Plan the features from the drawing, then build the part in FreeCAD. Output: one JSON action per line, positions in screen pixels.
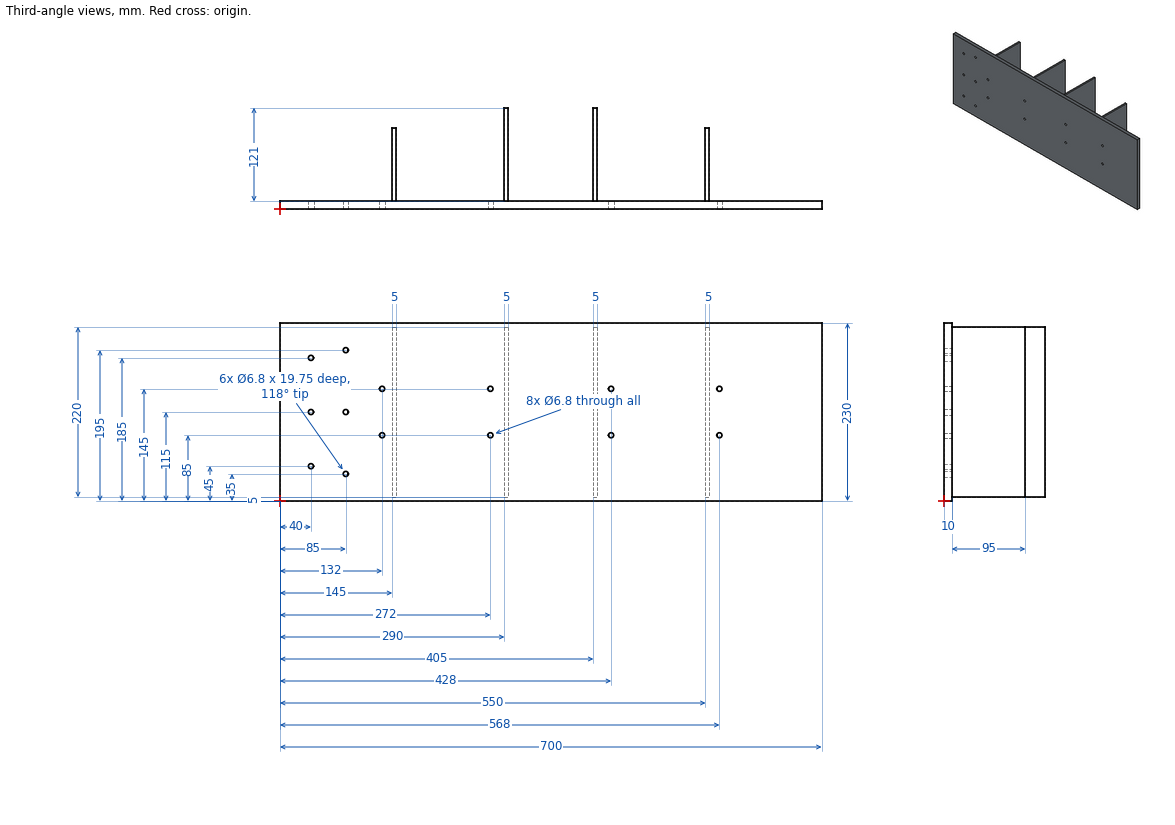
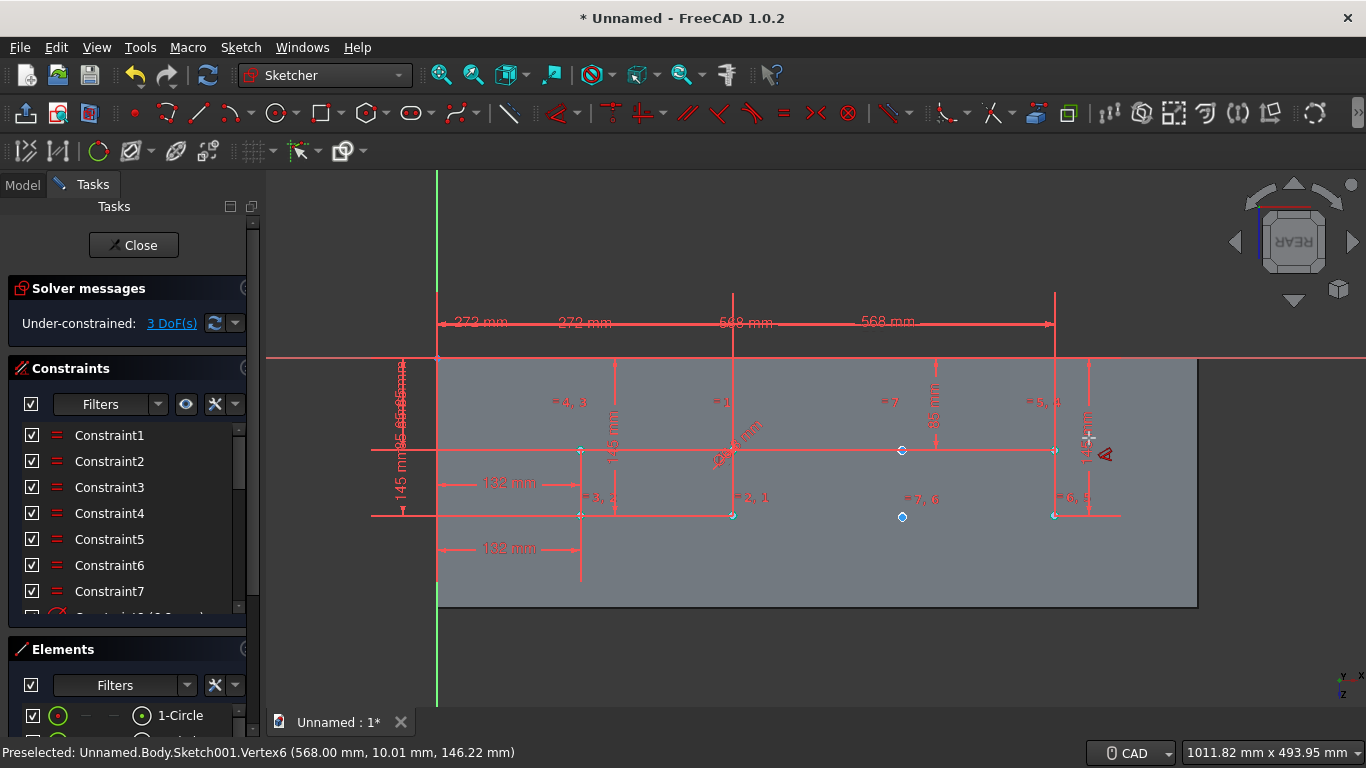
{"action": "left_click", "coordinate": [902, 517]}
{"action": "left_click", "coordinate": [670, 324]}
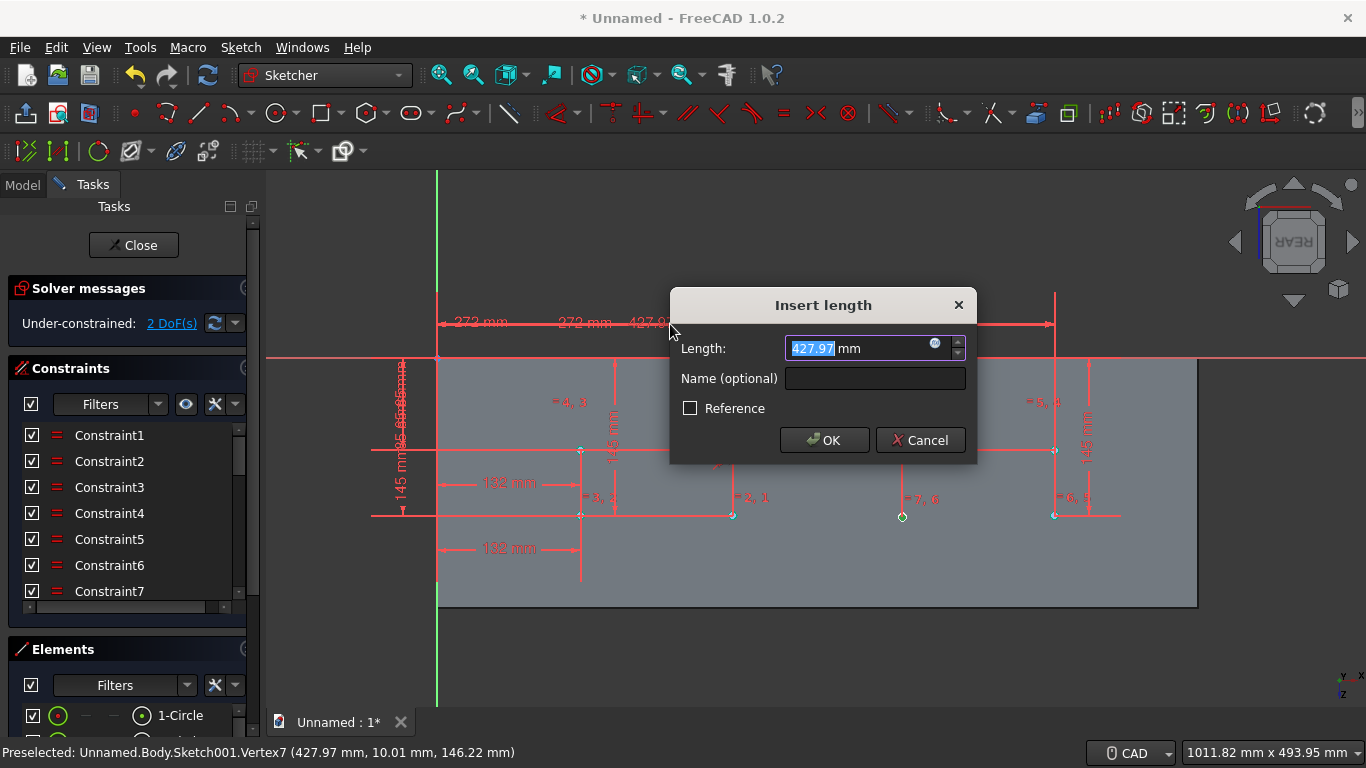
{"action": "type", "text": "428"}
{"action": "key", "text": "Return"}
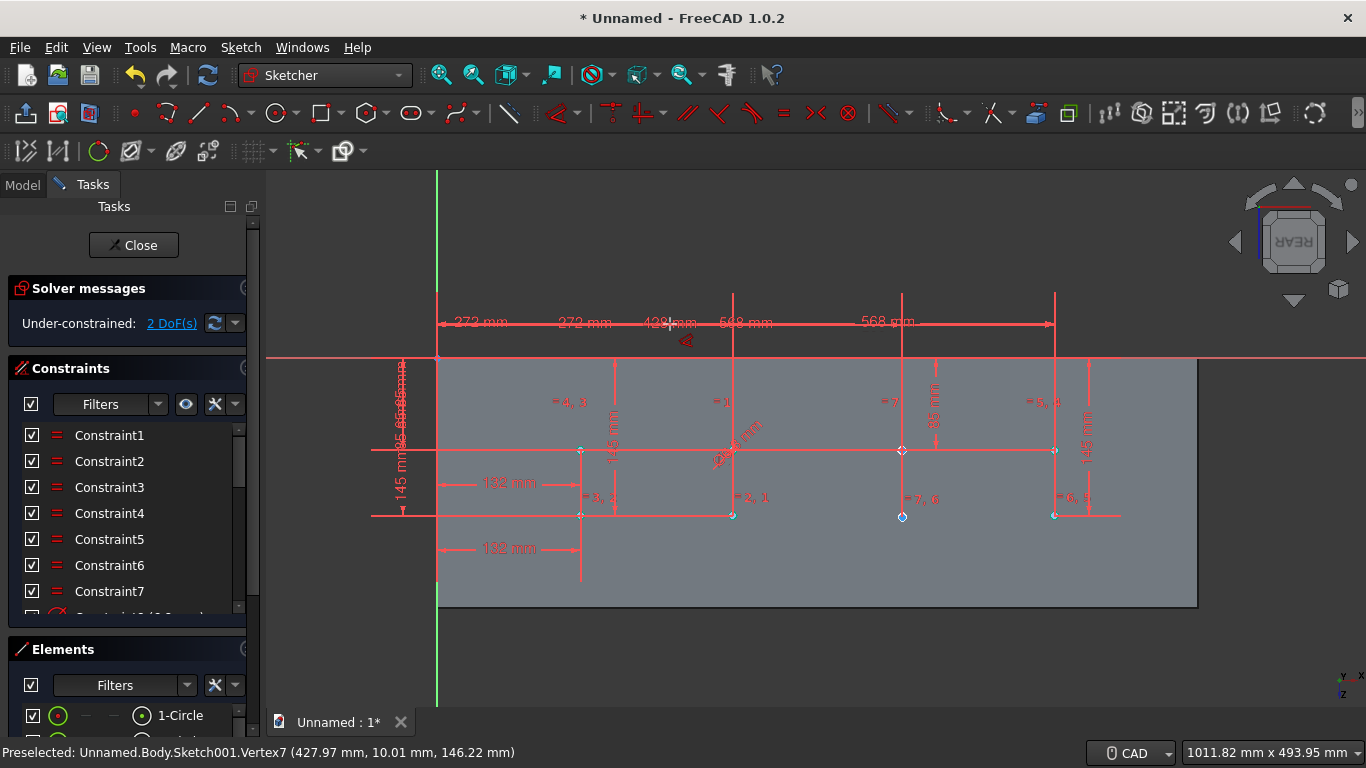
{"action": "left_click", "coordinate": [902, 517]}
{"action": "left_click", "coordinate": [936, 438]}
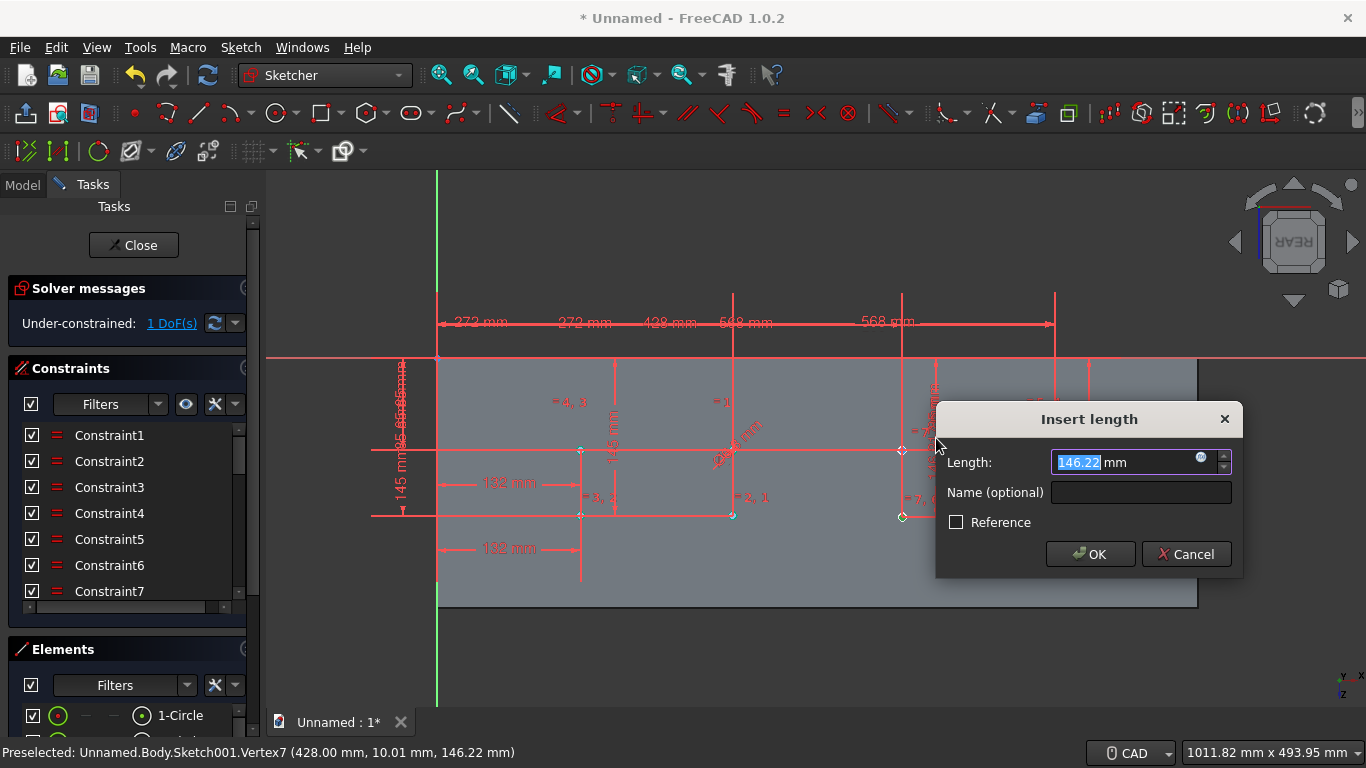
{"action": "type", "text": "145"}
{"action": "key", "text": "Return"}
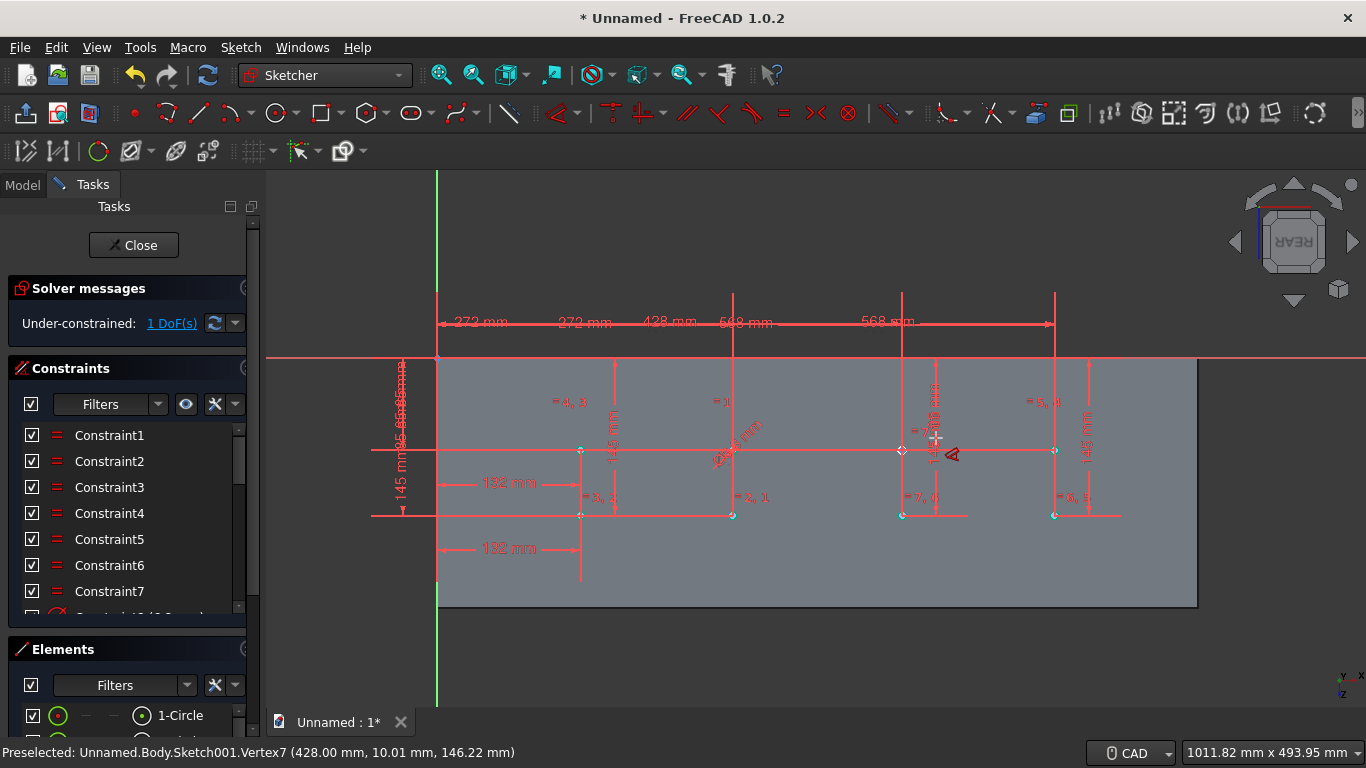
{"action": "left_click", "coordinate": [902, 450]}
{"action": "left_click", "coordinate": [670, 484]}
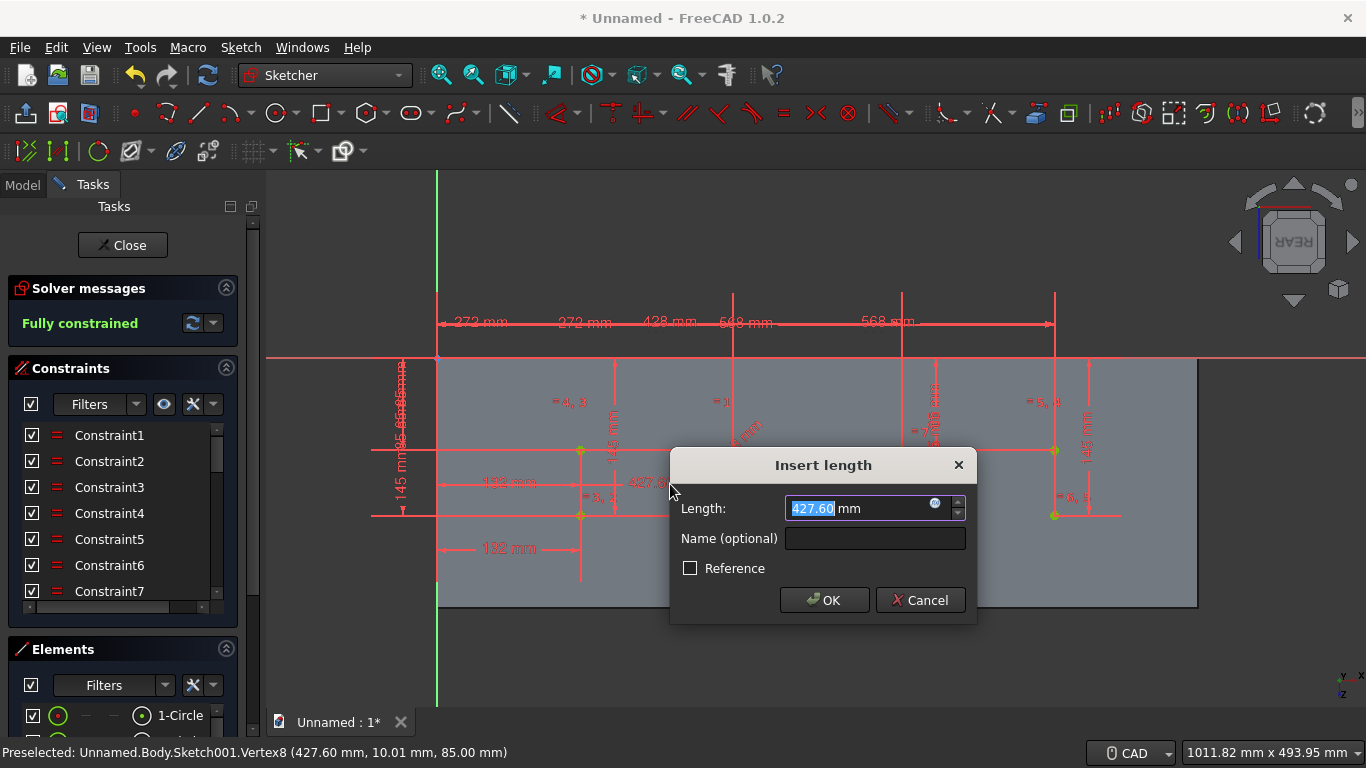
{"action": "type", "text": "428"}
{"action": "key", "text": "Return"}
{"action": "key", "text": "Escape"}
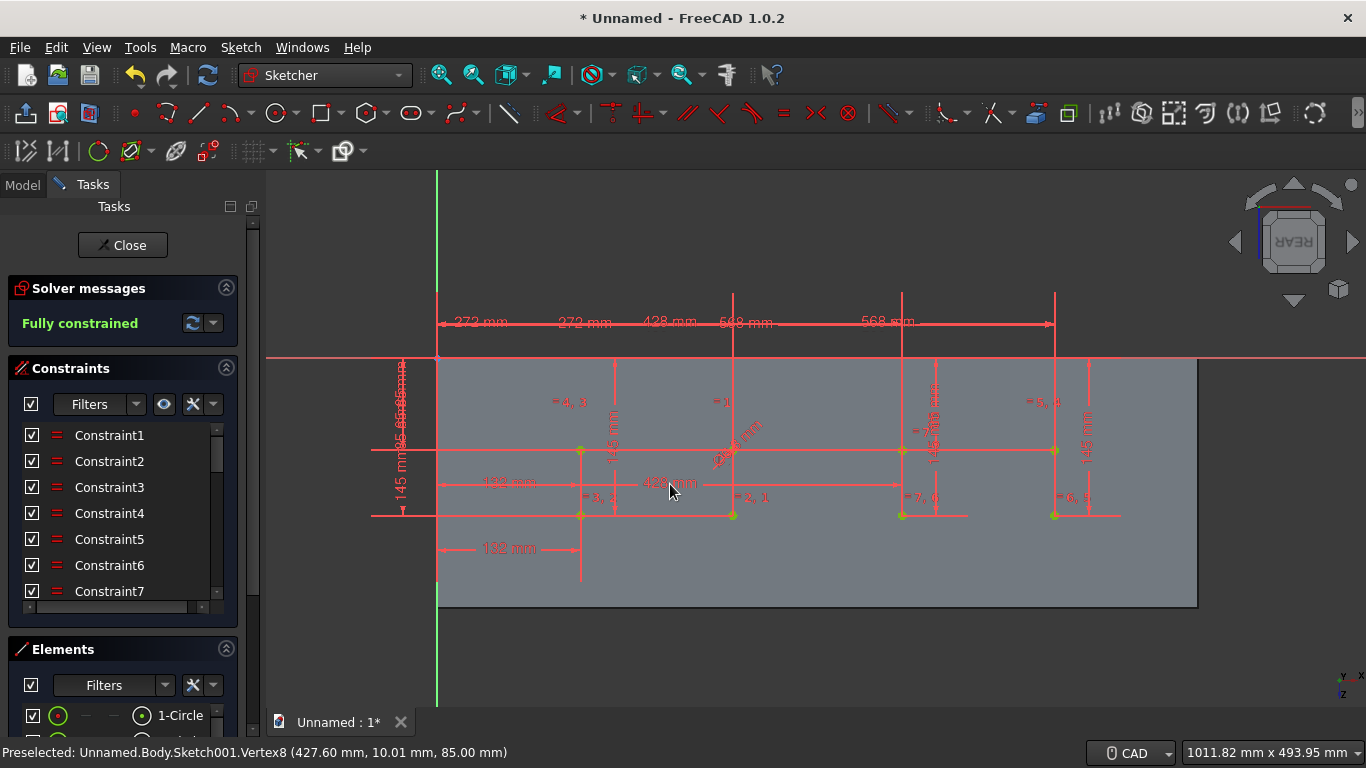
{"action": "left_click", "coordinate": [123, 245]}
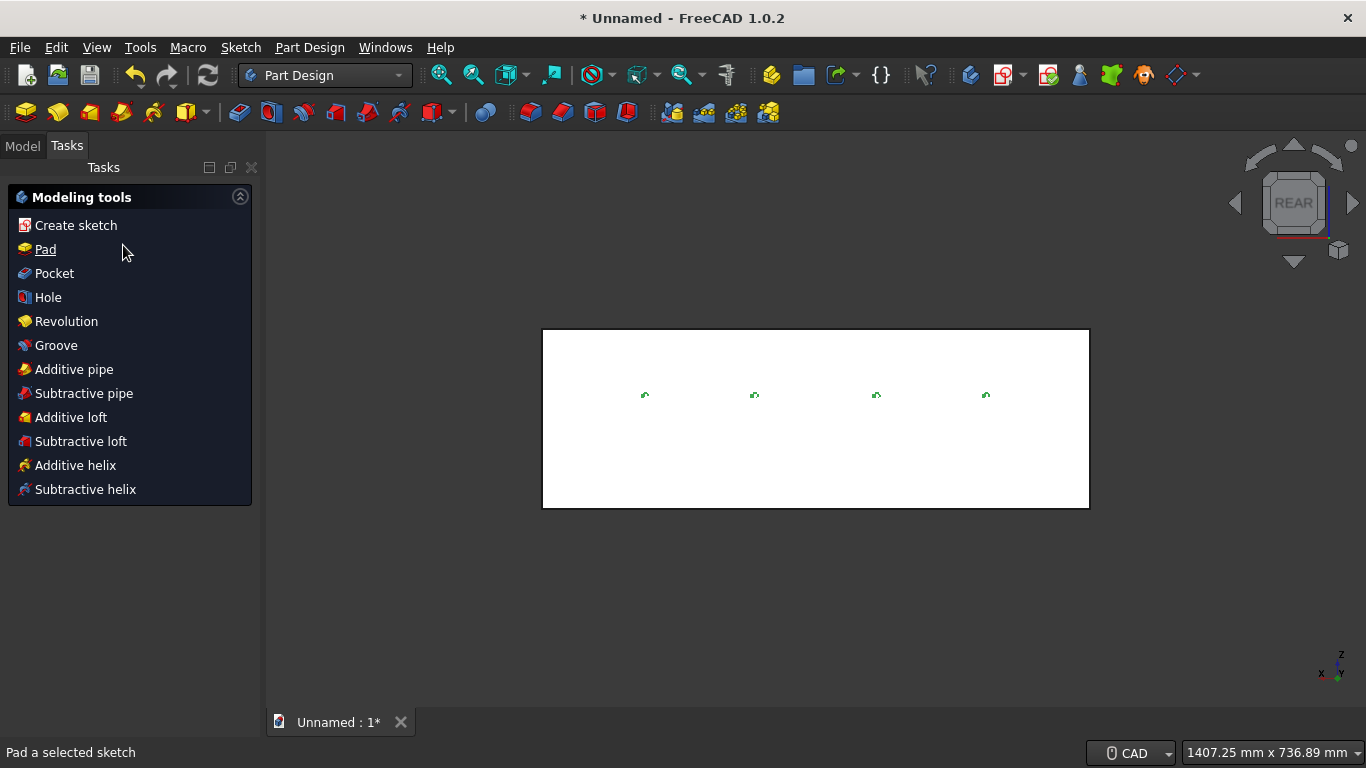
{"action": "left_click", "coordinate": [272, 112]}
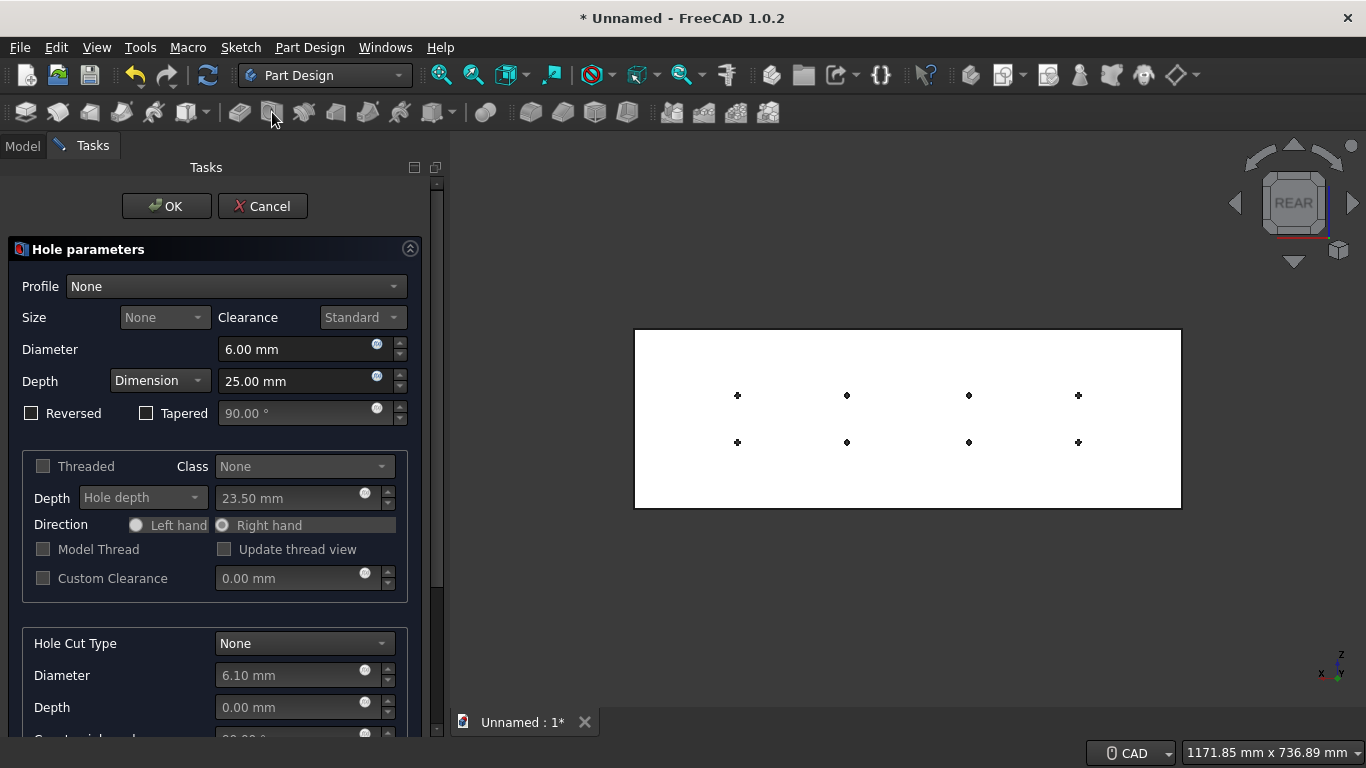
{"action": "triple_click", "coordinate": [305, 349]}